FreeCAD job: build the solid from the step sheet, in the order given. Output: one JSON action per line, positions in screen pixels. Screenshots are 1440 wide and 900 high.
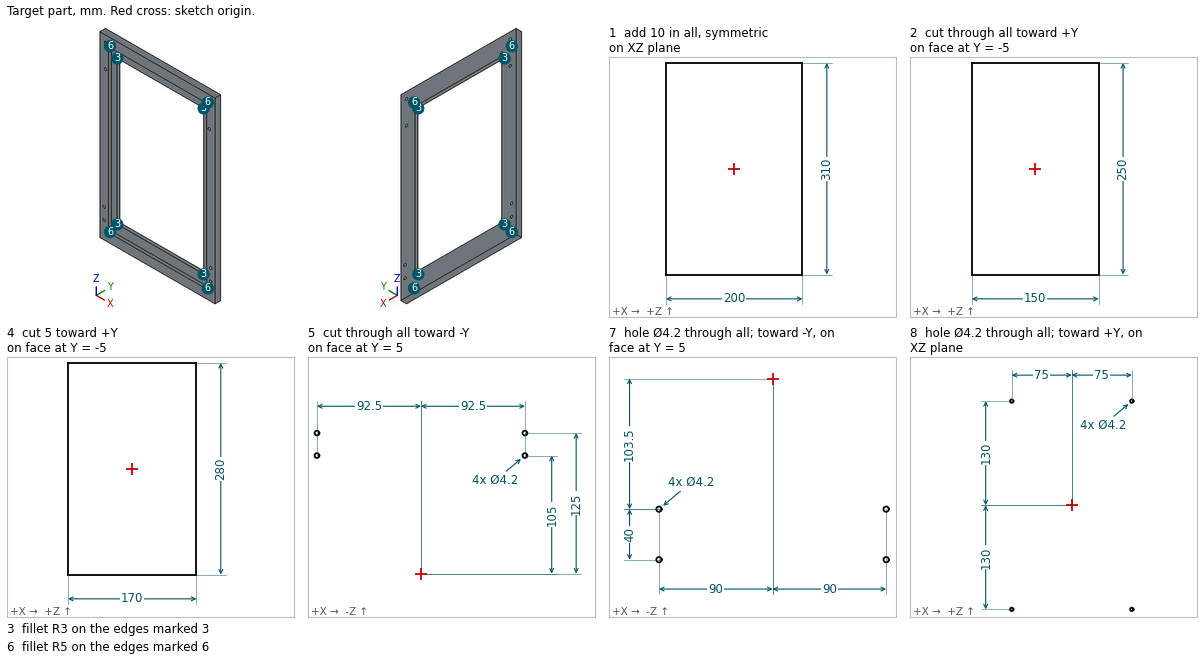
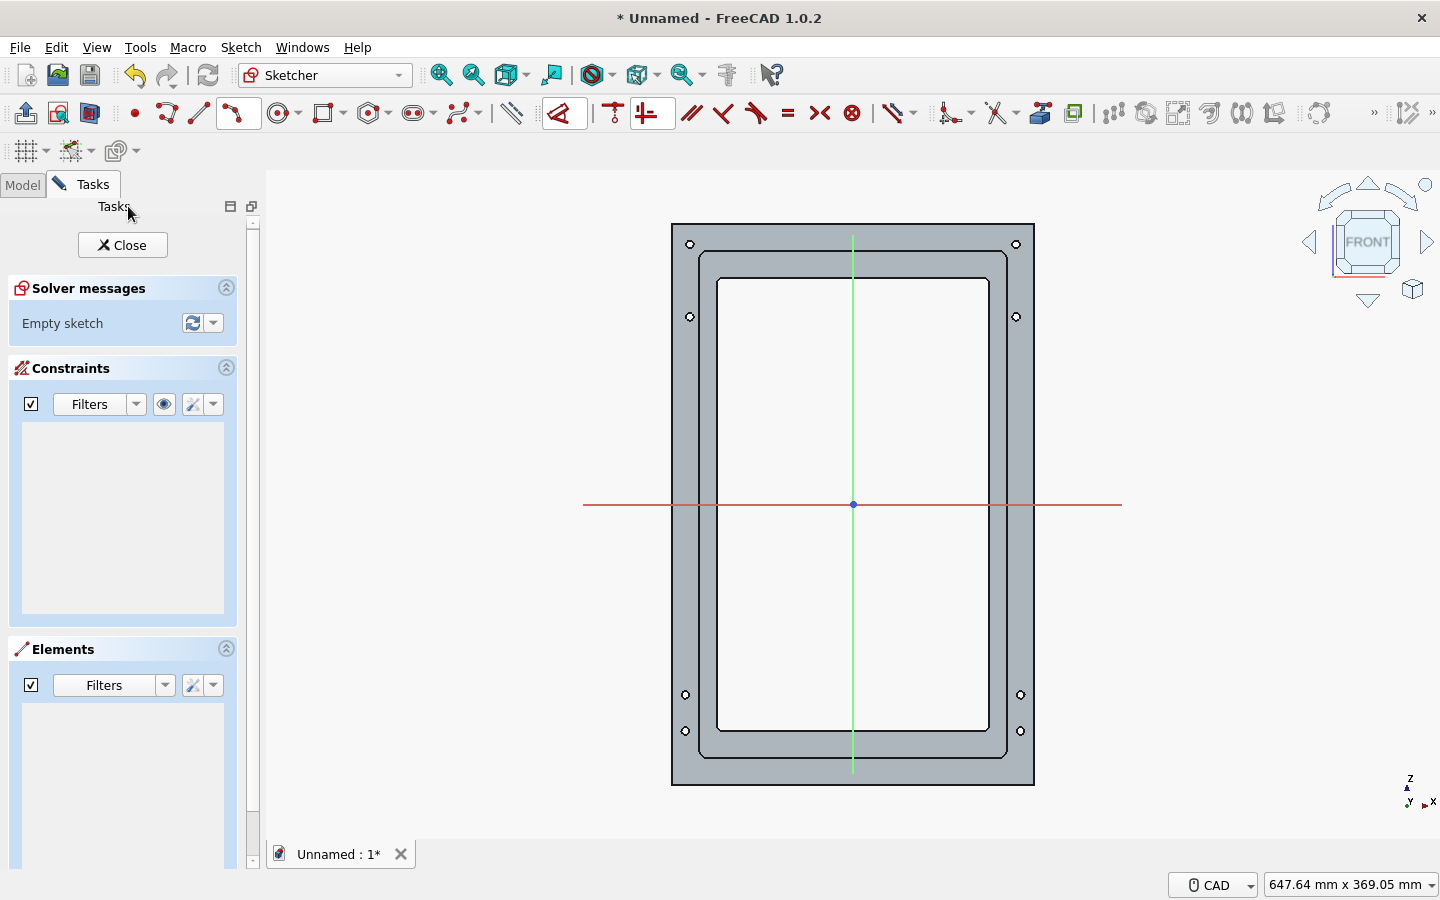
{"action": "key", "text": "g c"}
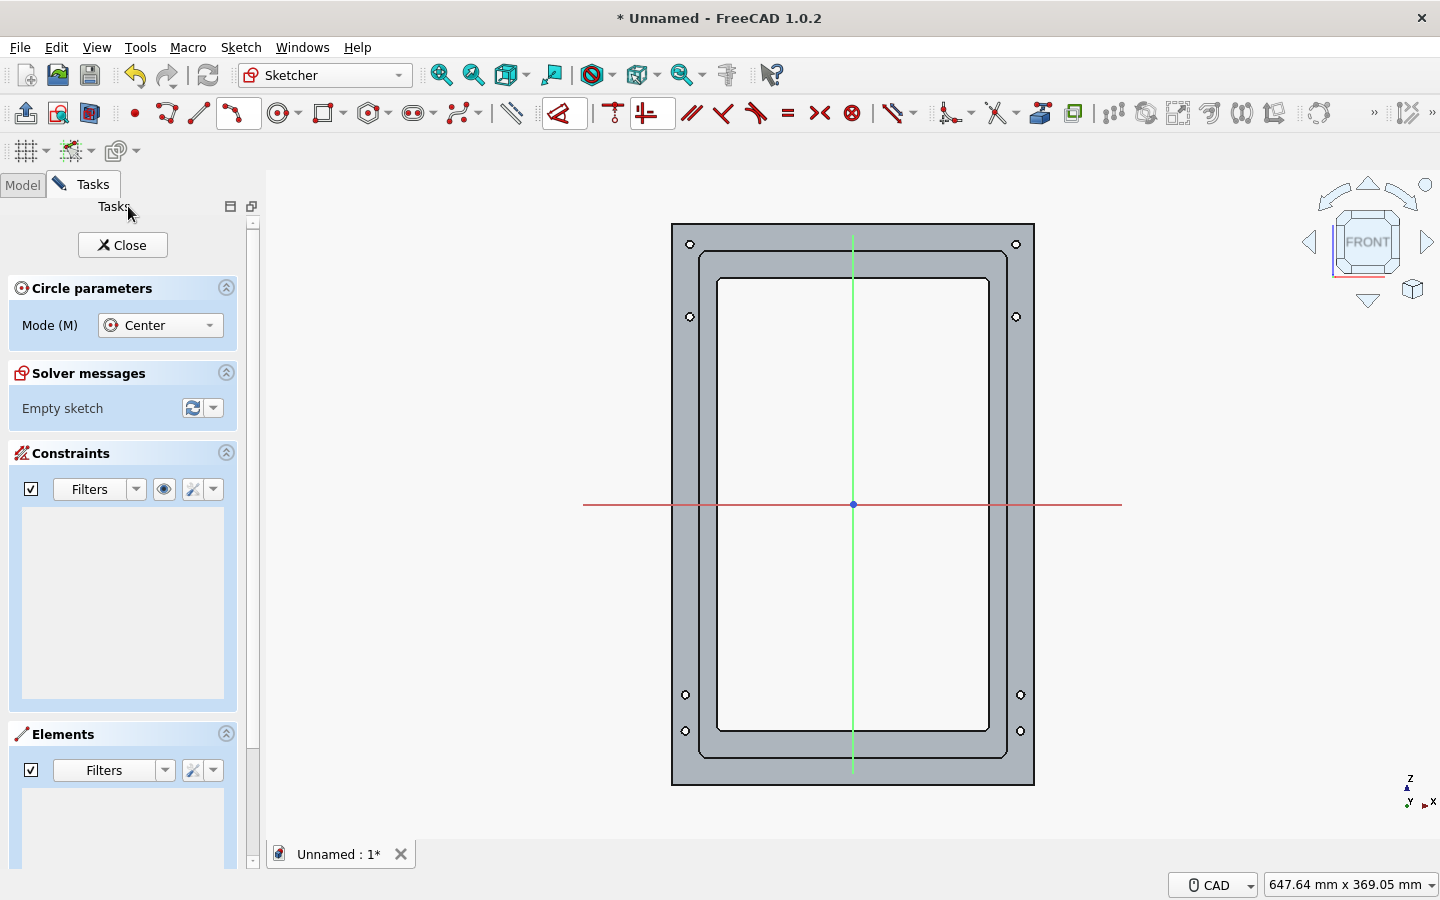
{"action": "scroll", "coordinate": [717, 269], "scroll_direction": "up", "scroll_amount": 9}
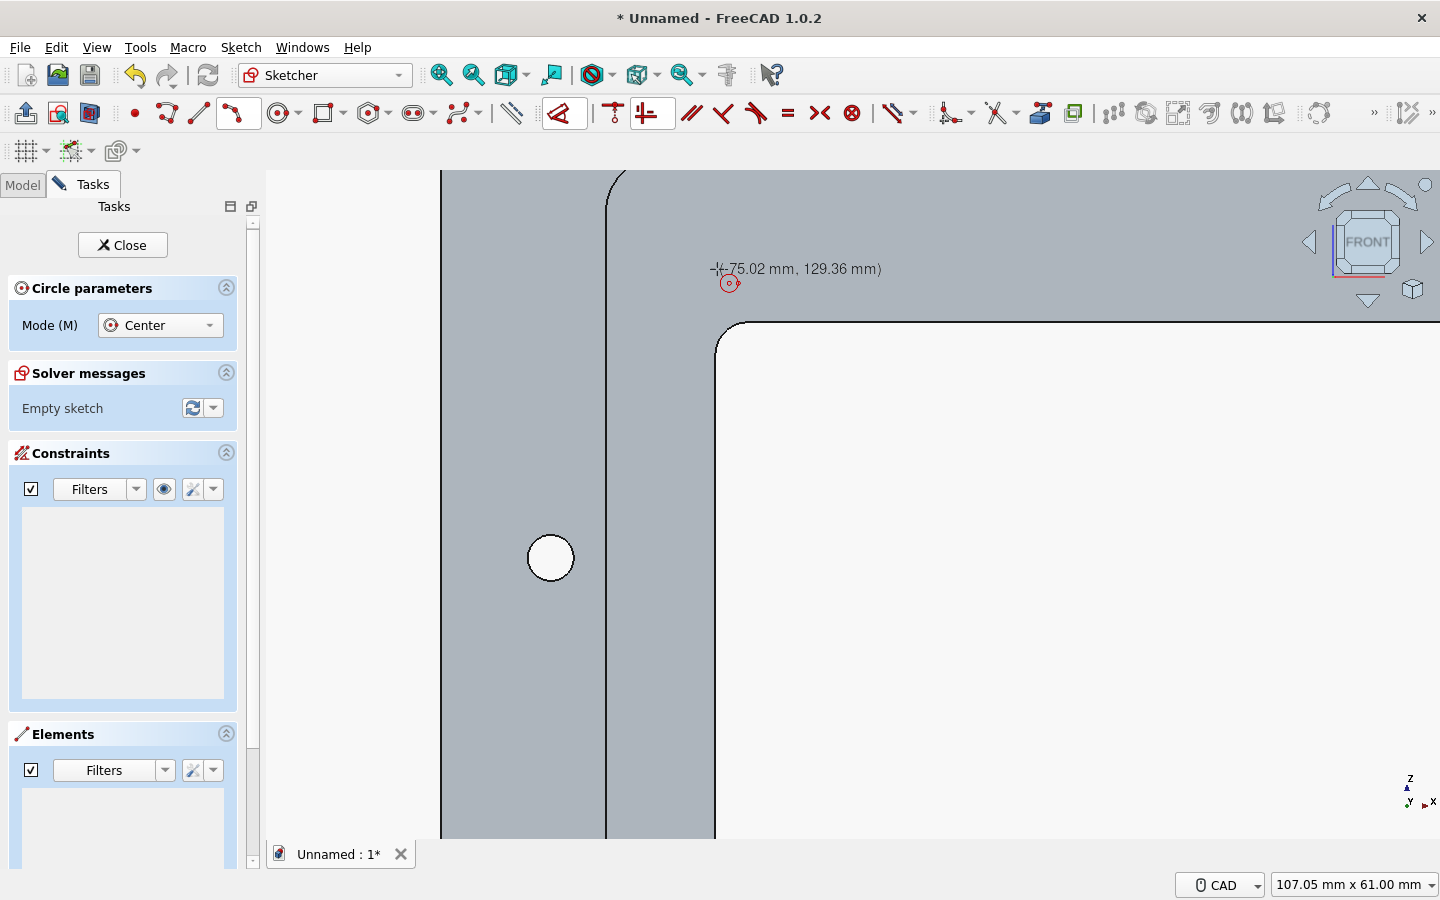
{"action": "scroll", "coordinate": [667, 318], "scroll_direction": "down", "scroll_amount": 10}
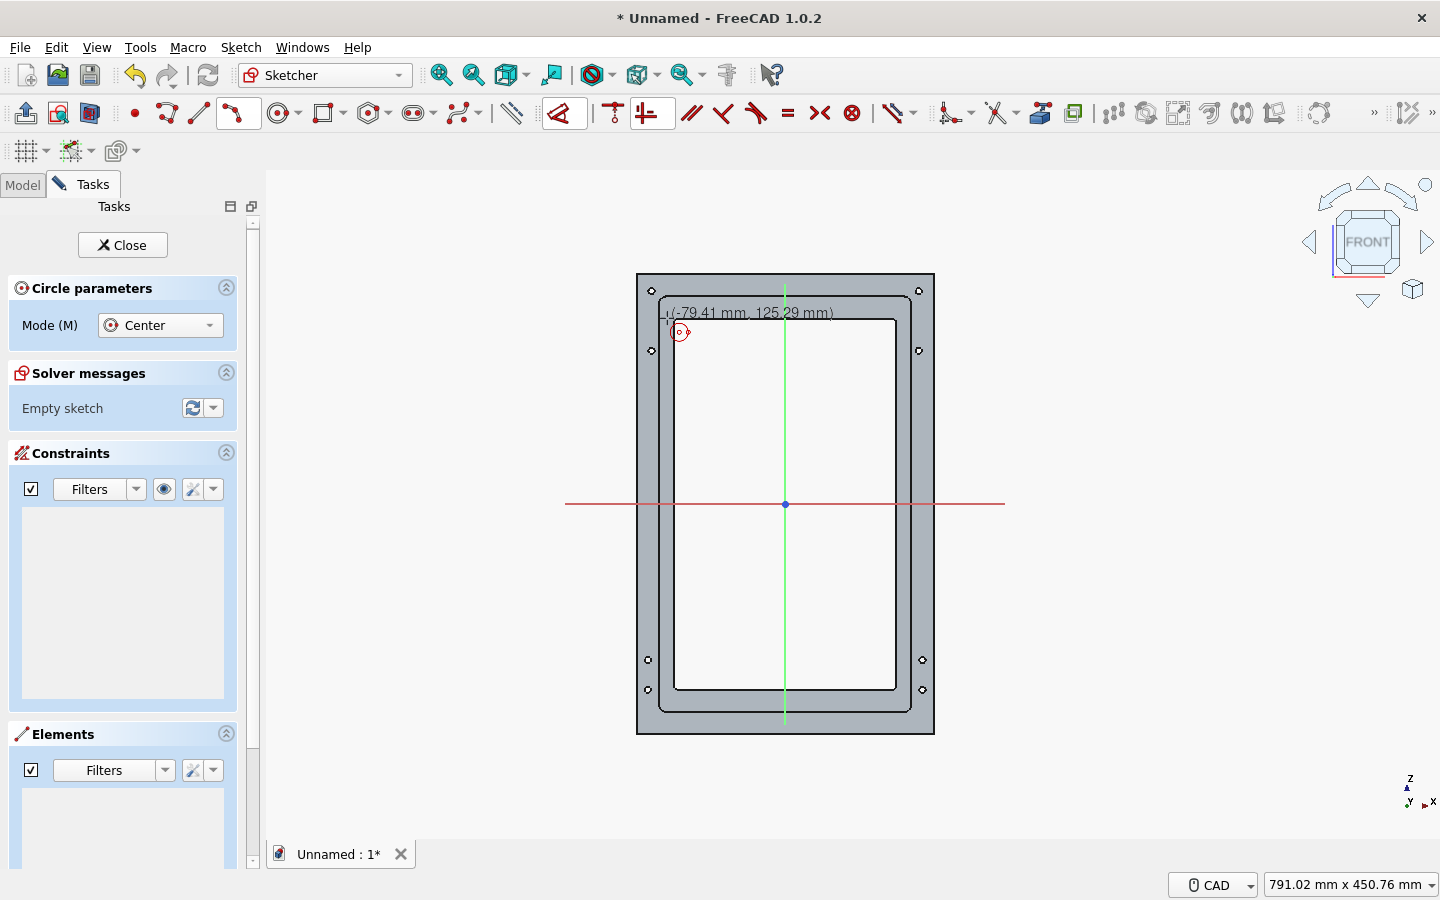
{"action": "left_click", "coordinate": [674, 311]}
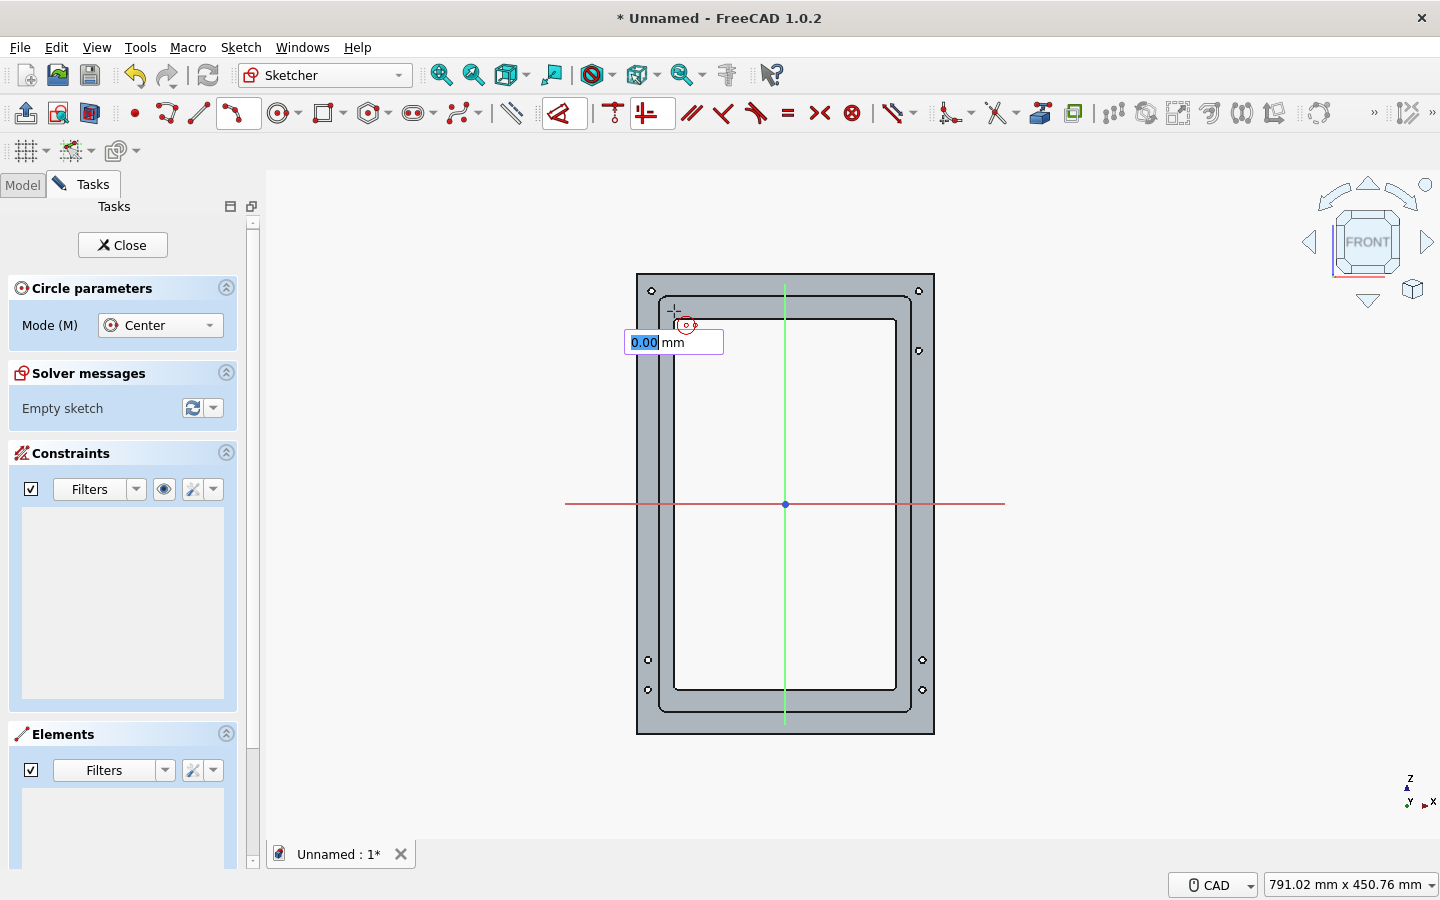
{"action": "scroll", "coordinate": [676, 309], "scroll_direction": "up", "scroll_amount": 9}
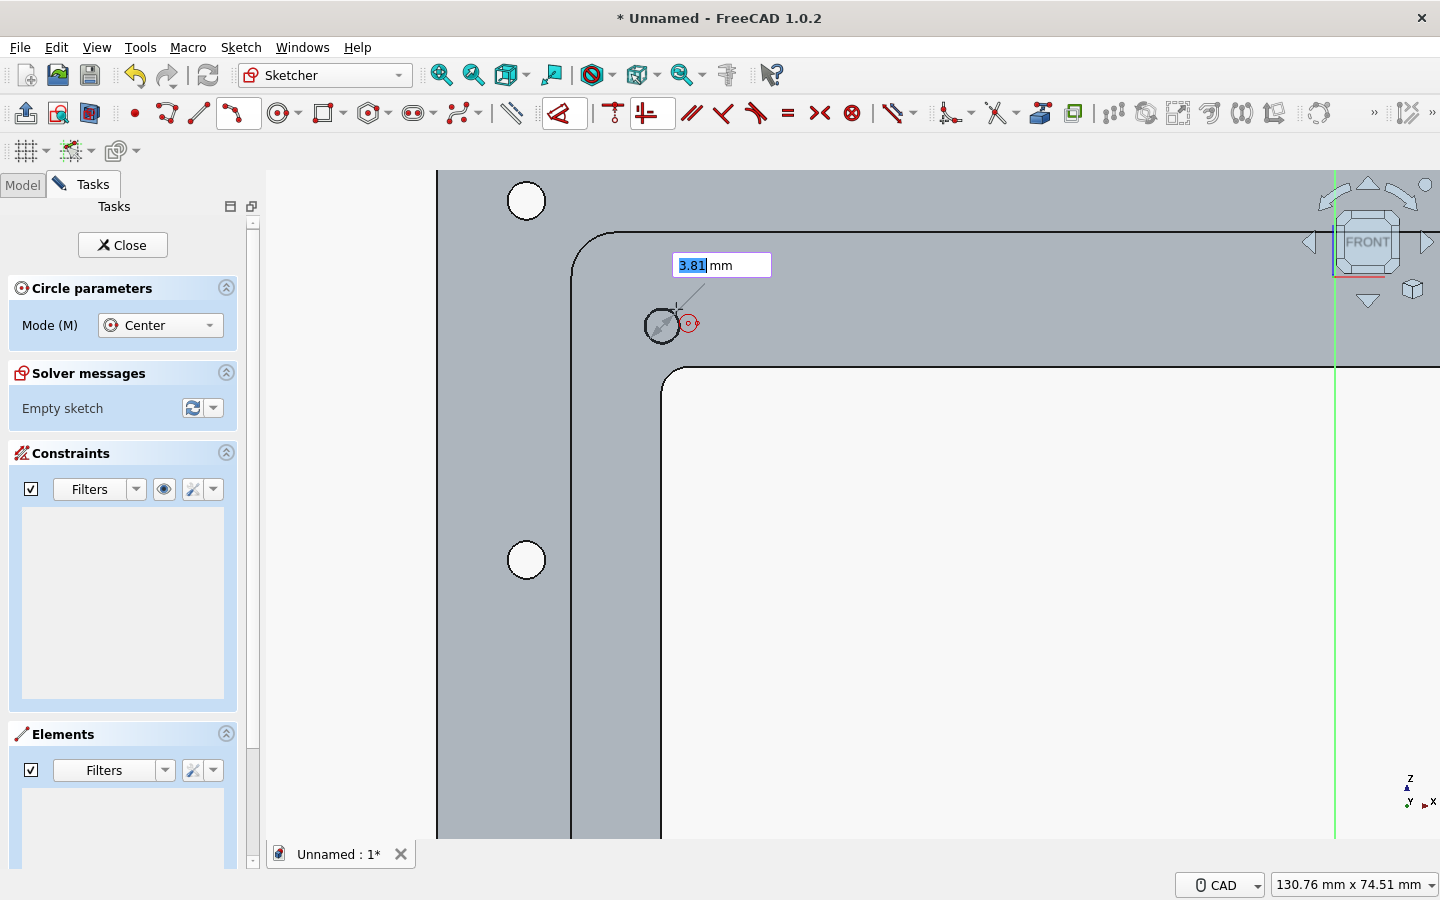
{"action": "left_click", "coordinate": [674, 309]}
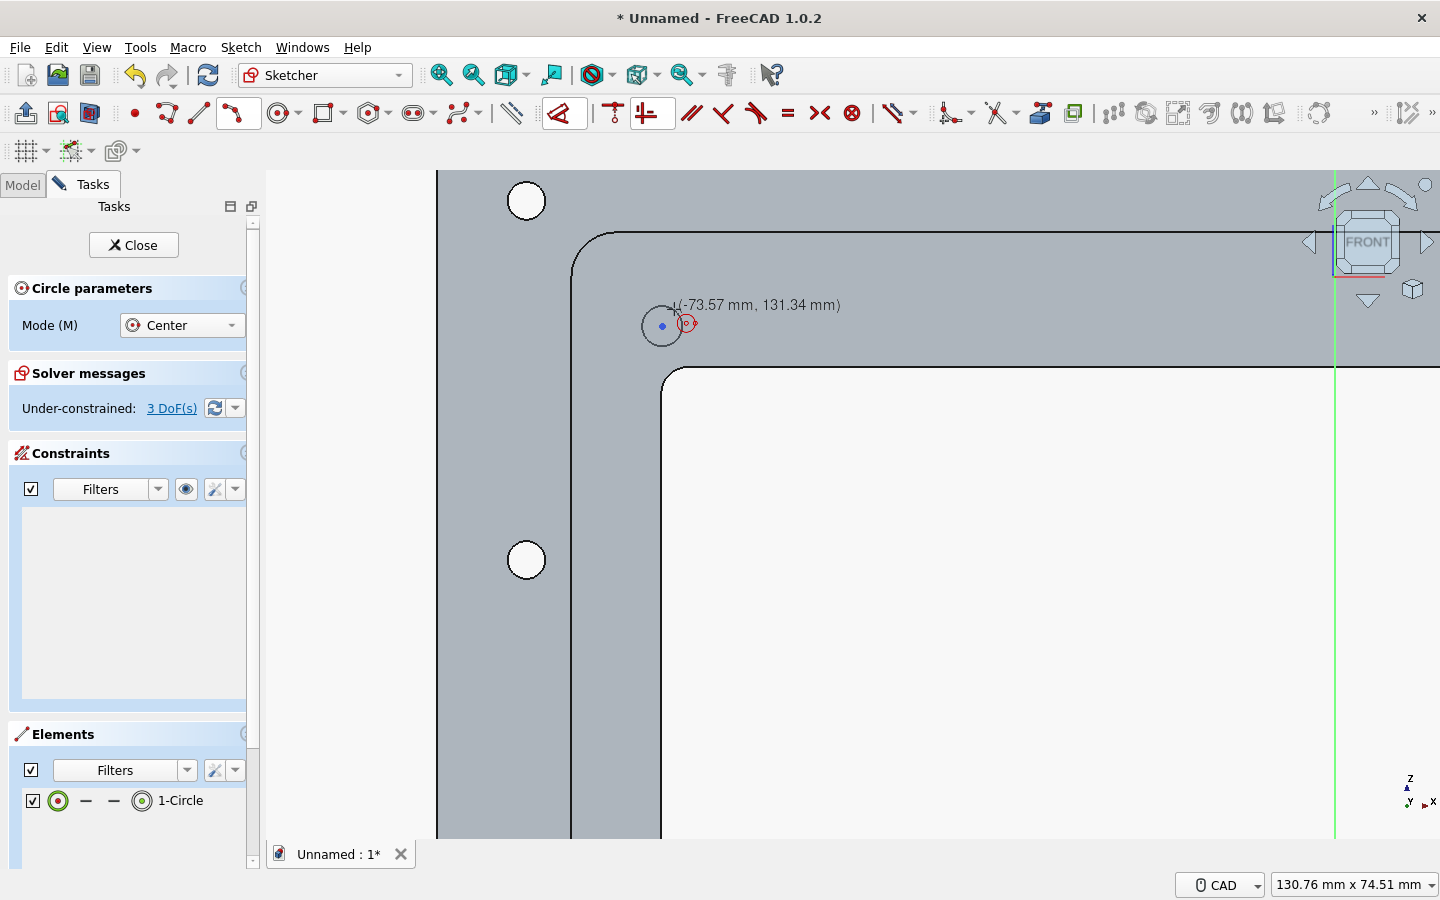
{"action": "scroll", "coordinate": [676, 309], "scroll_direction": "down", "scroll_amount": 9}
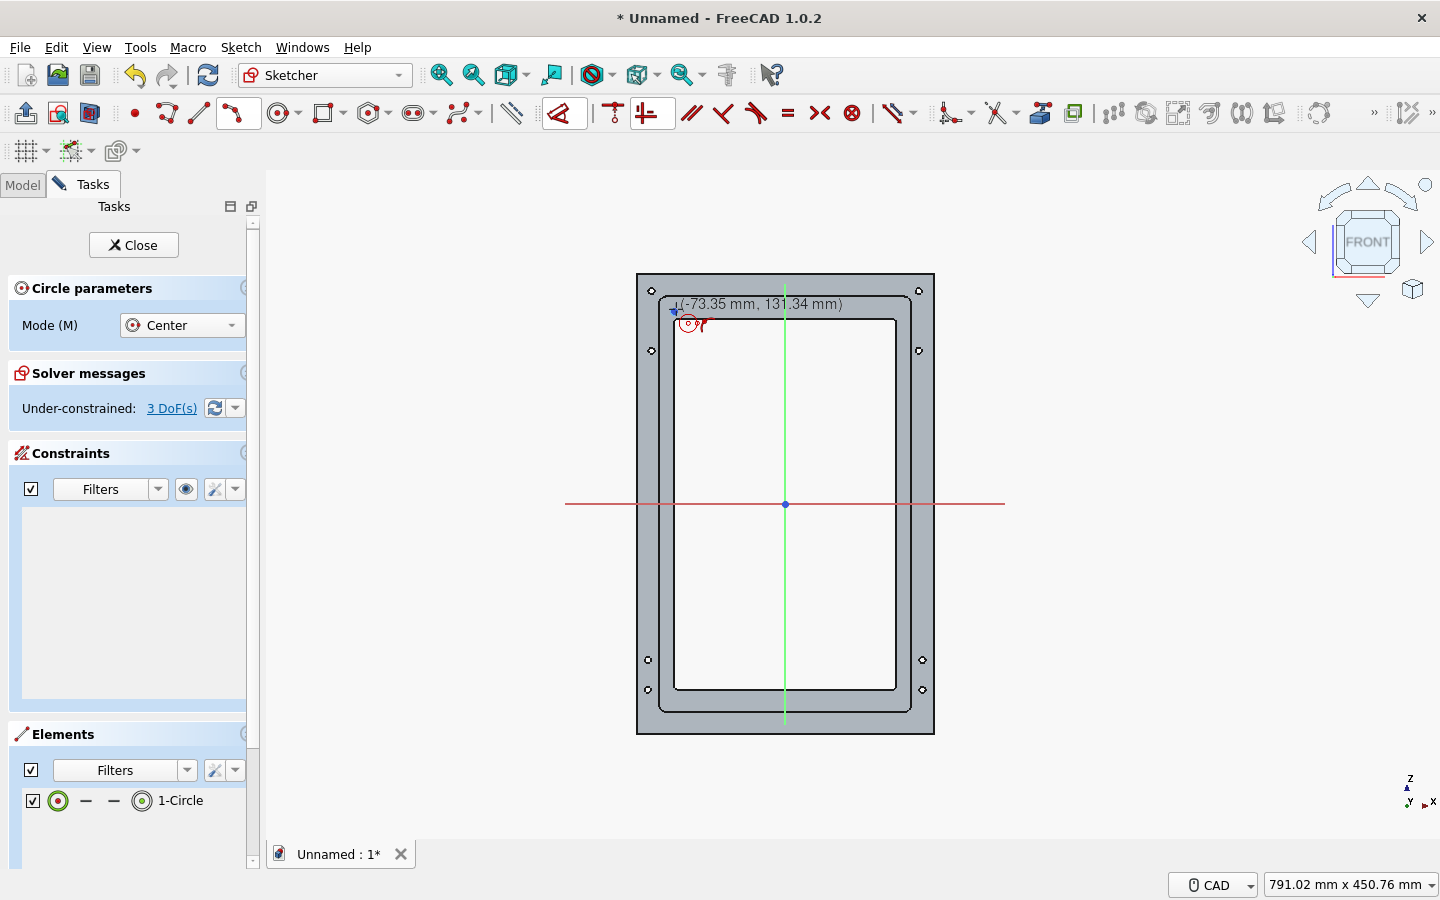
{"action": "scroll", "coordinate": [896, 311], "scroll_direction": "up", "scroll_amount": 10}